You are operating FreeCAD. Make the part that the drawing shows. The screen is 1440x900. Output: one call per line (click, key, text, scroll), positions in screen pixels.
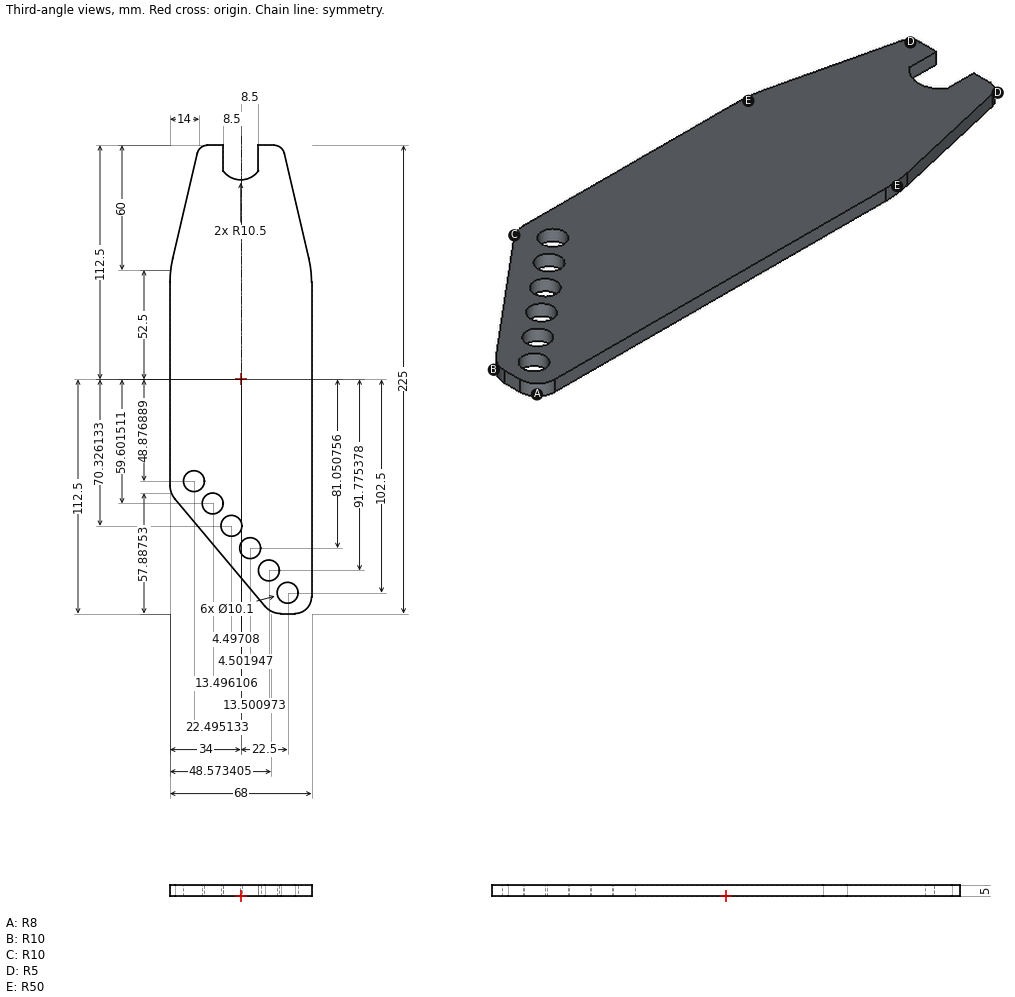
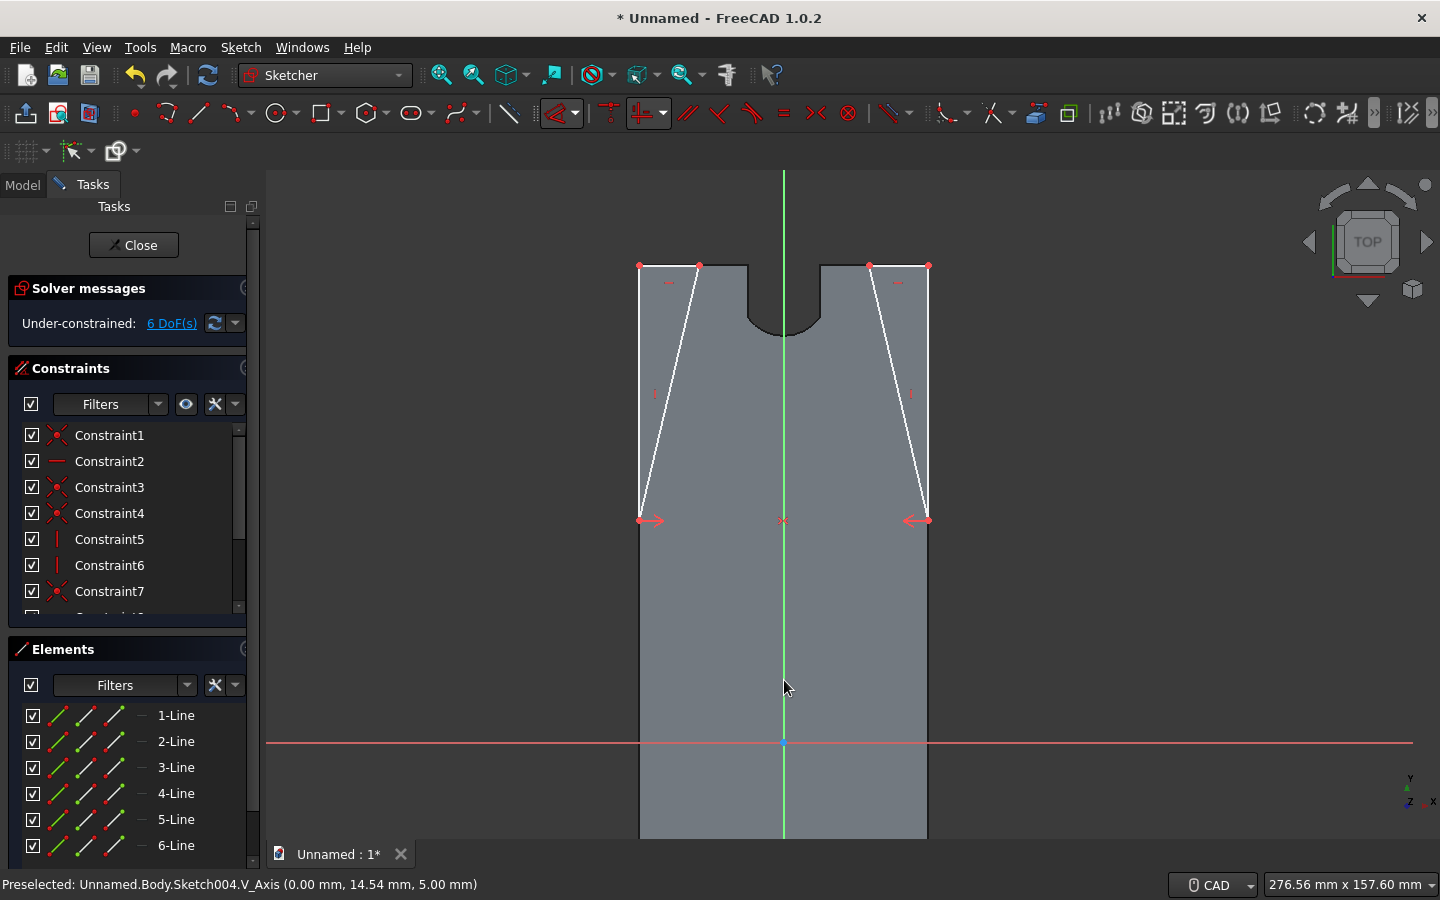
click(699, 266)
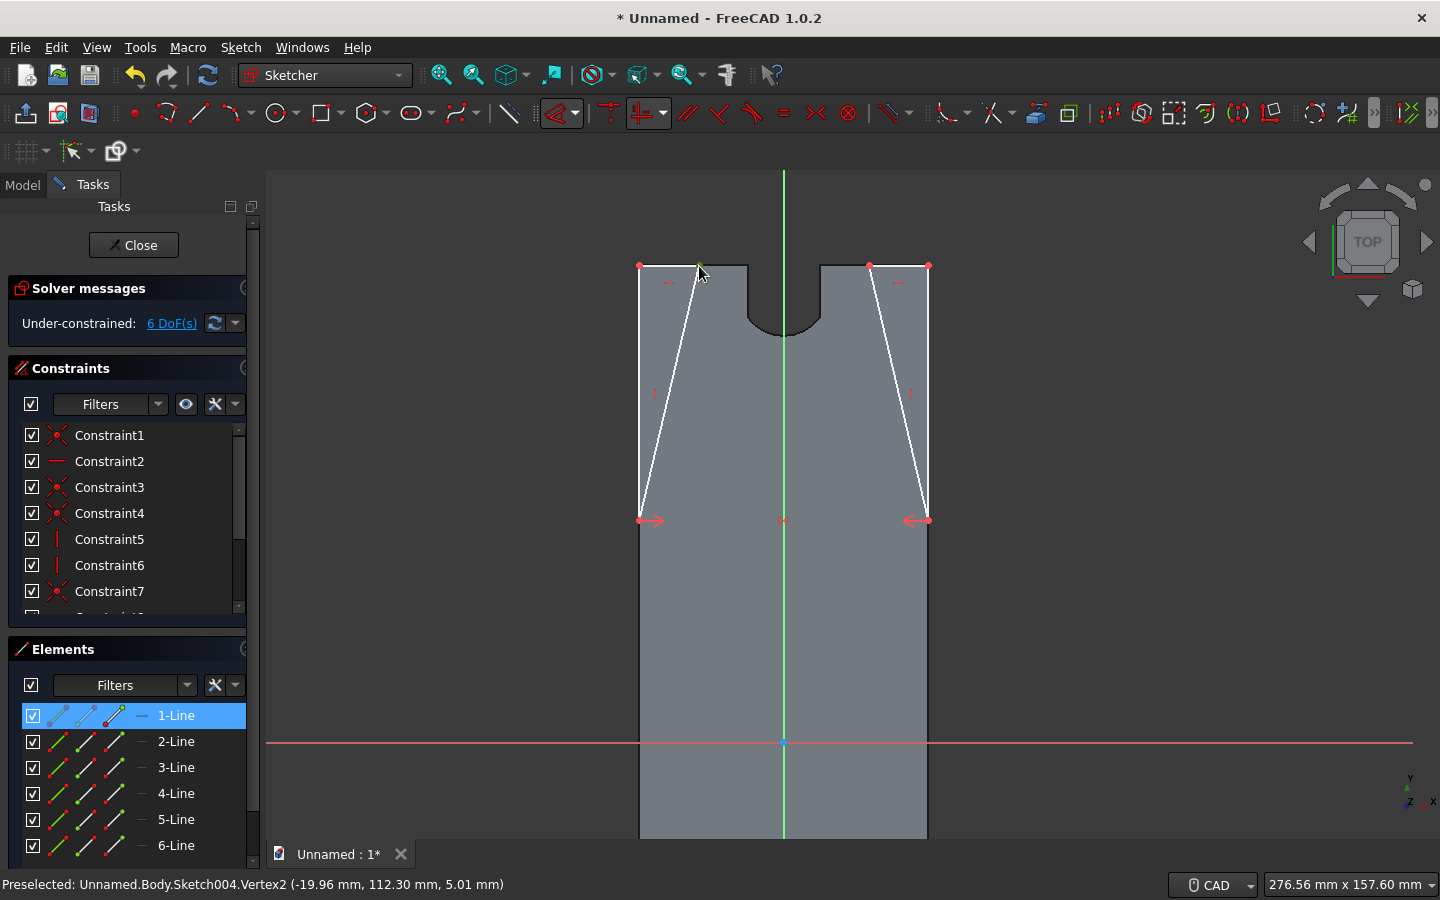
click(869, 266)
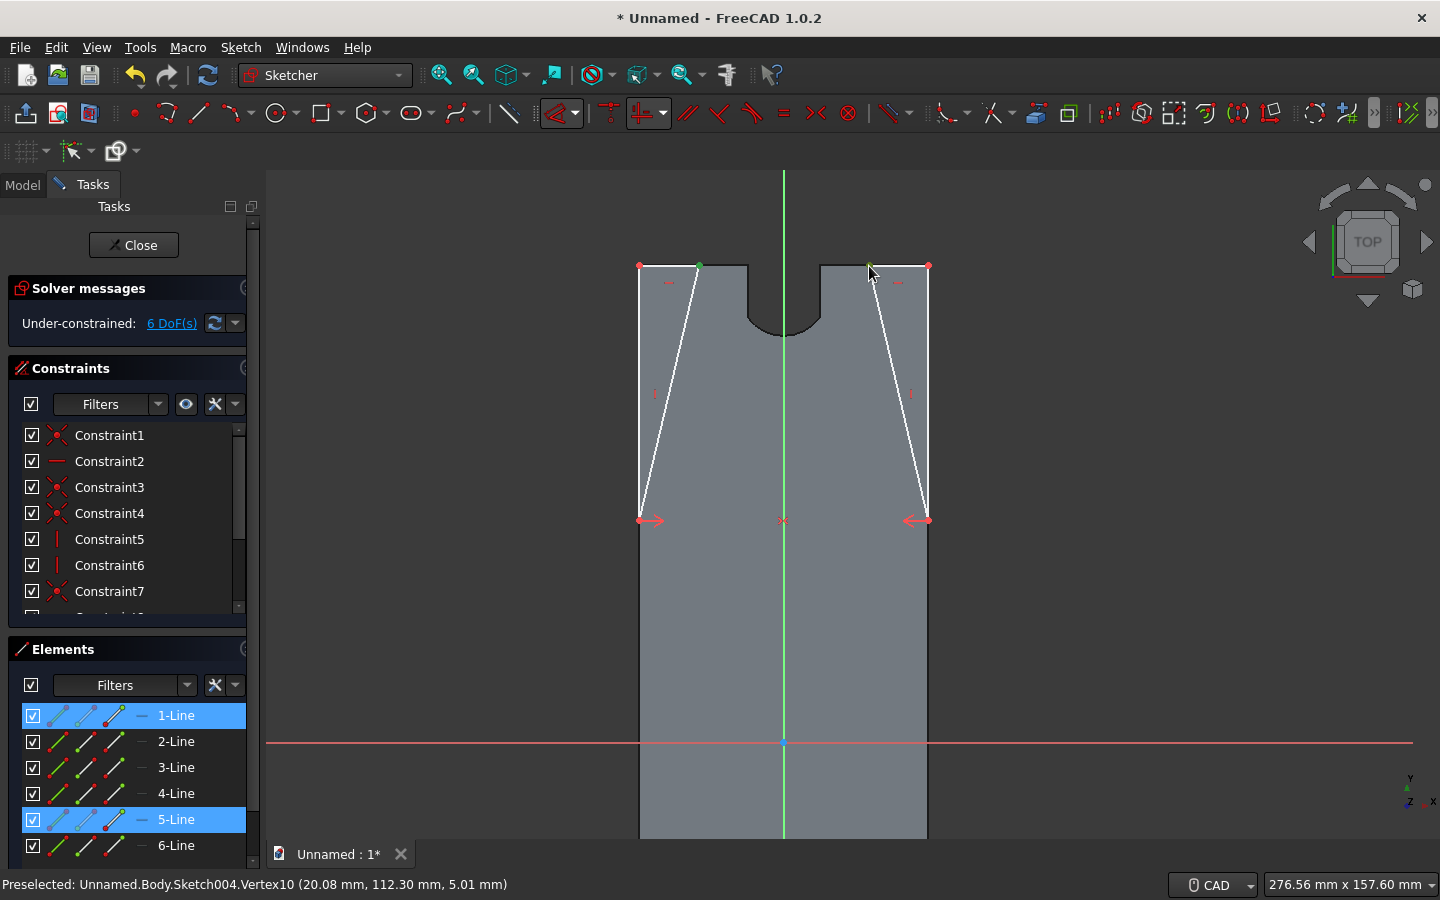
click(784, 680)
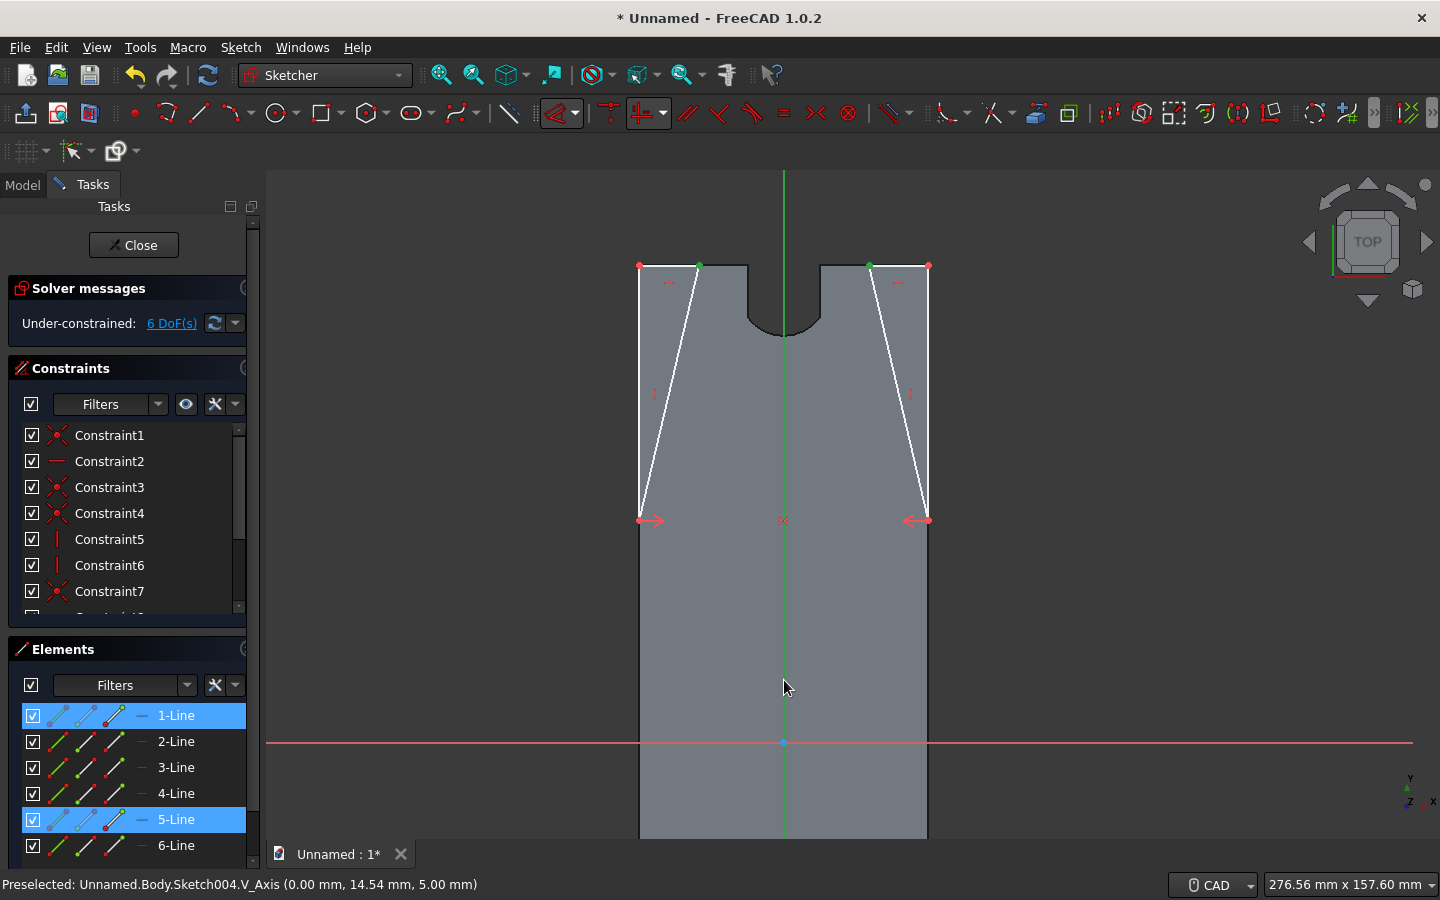
key(s)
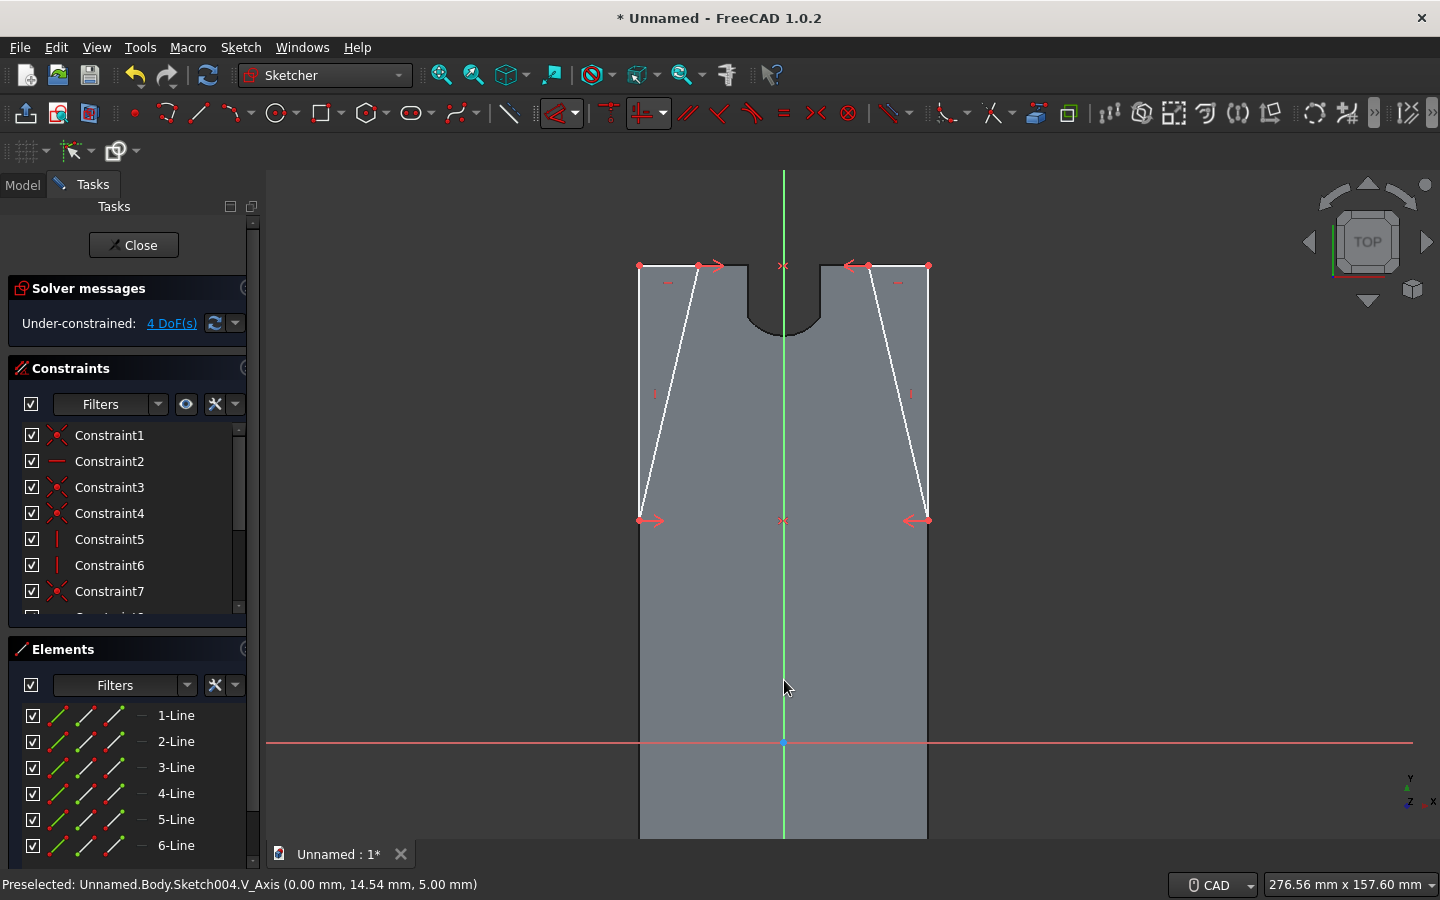
click(681, 266)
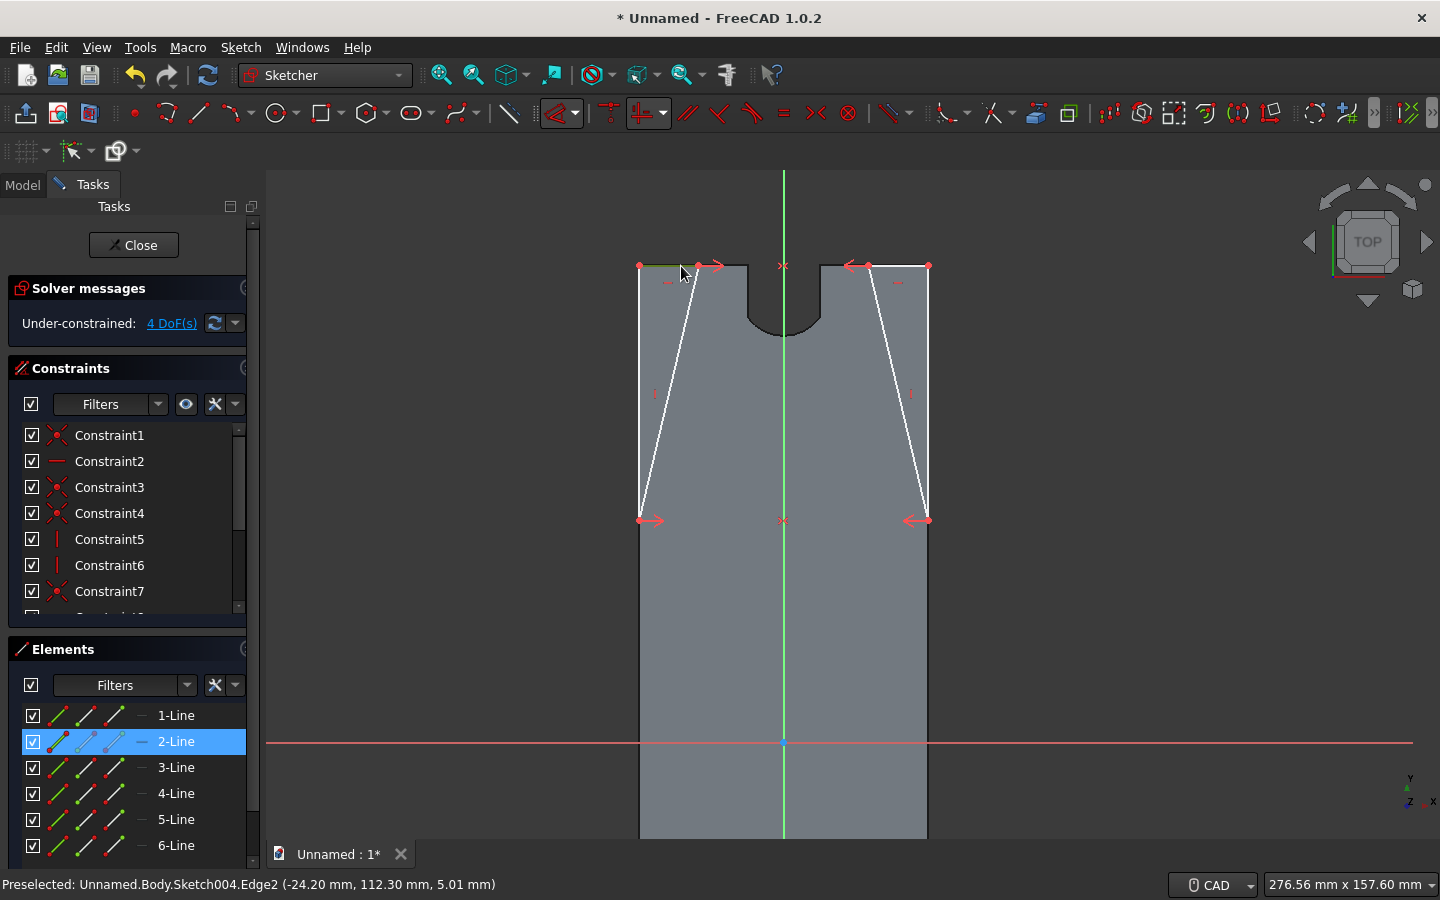
key(l)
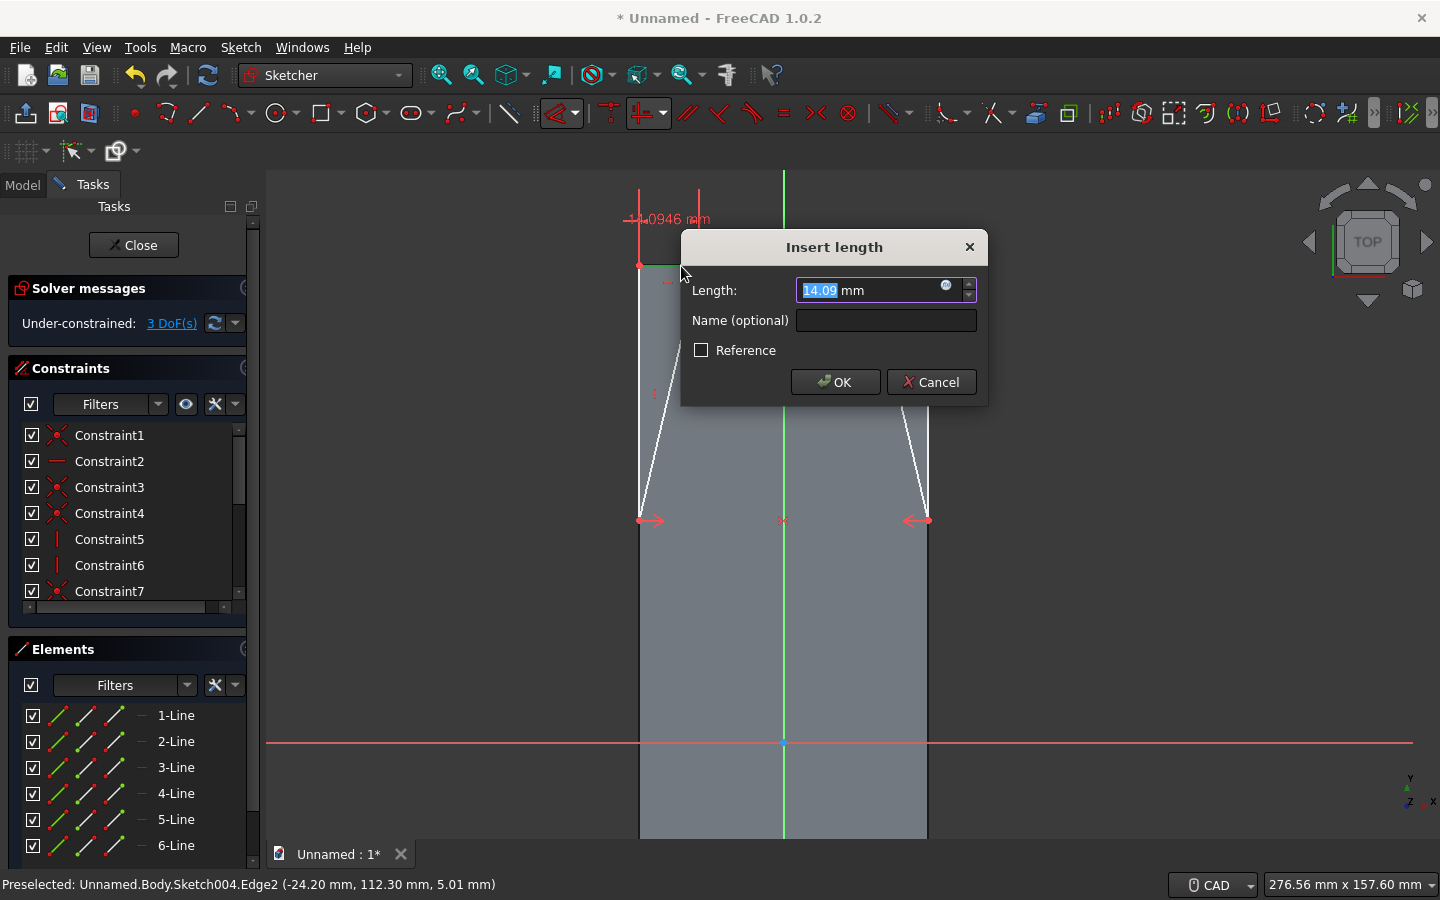
text(14)
key(Return)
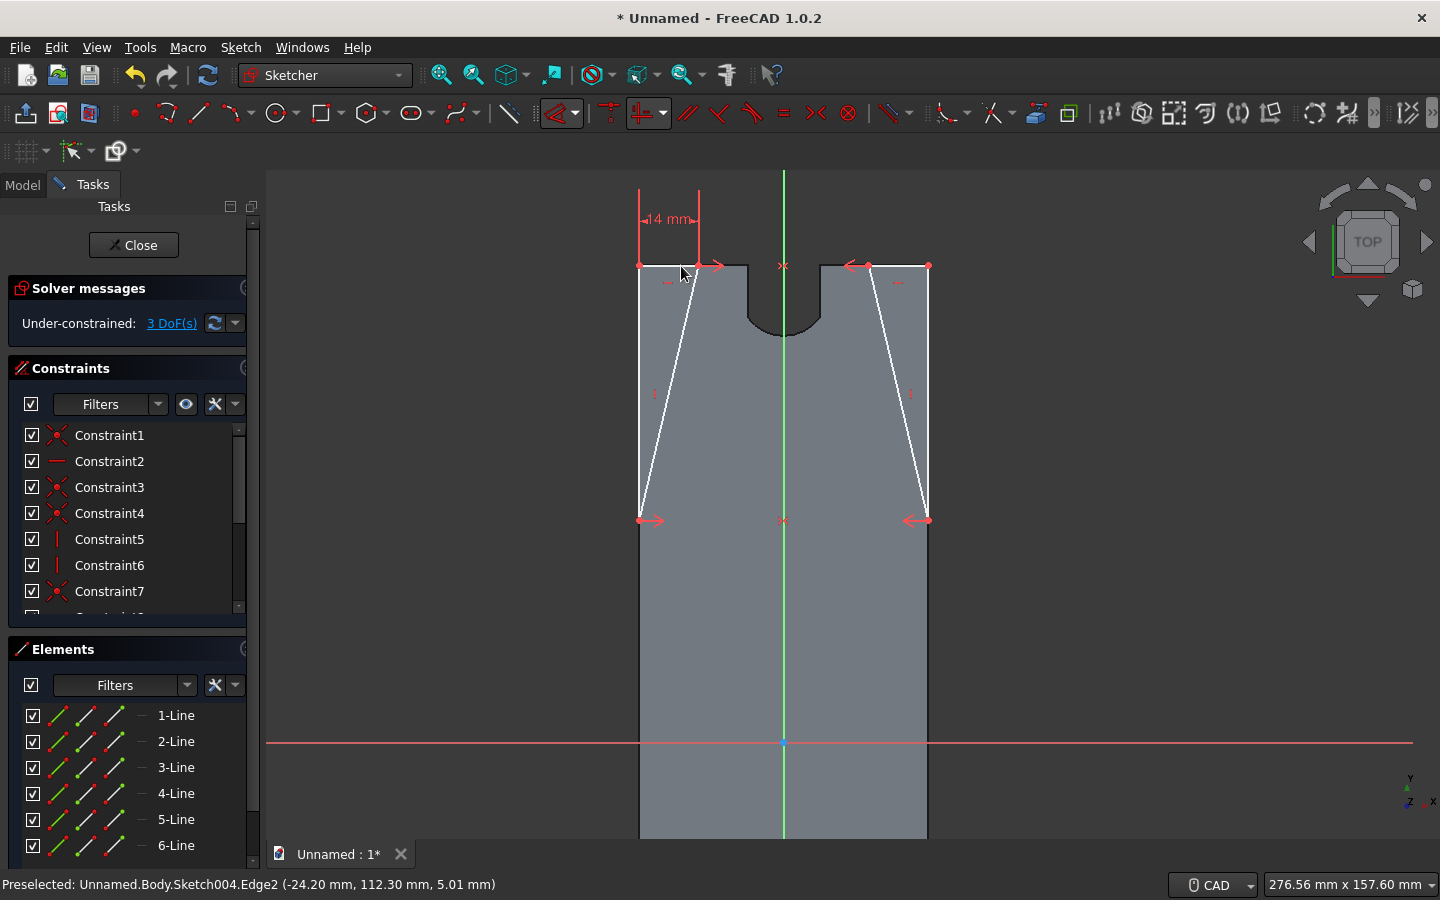
click(639, 342)